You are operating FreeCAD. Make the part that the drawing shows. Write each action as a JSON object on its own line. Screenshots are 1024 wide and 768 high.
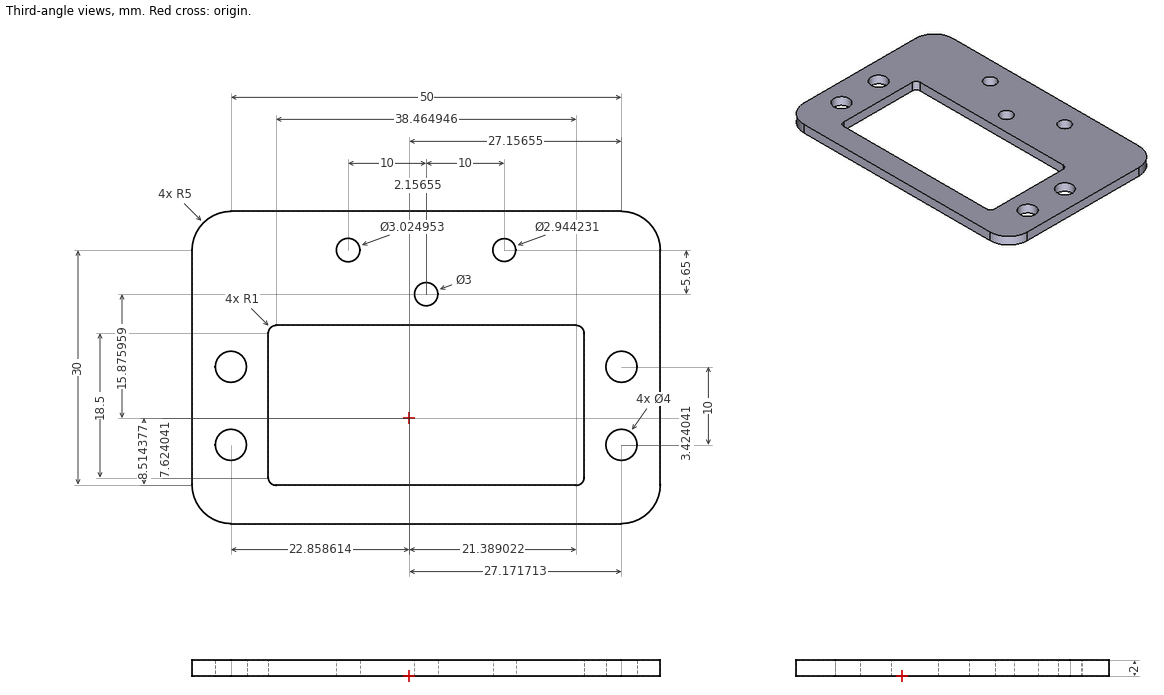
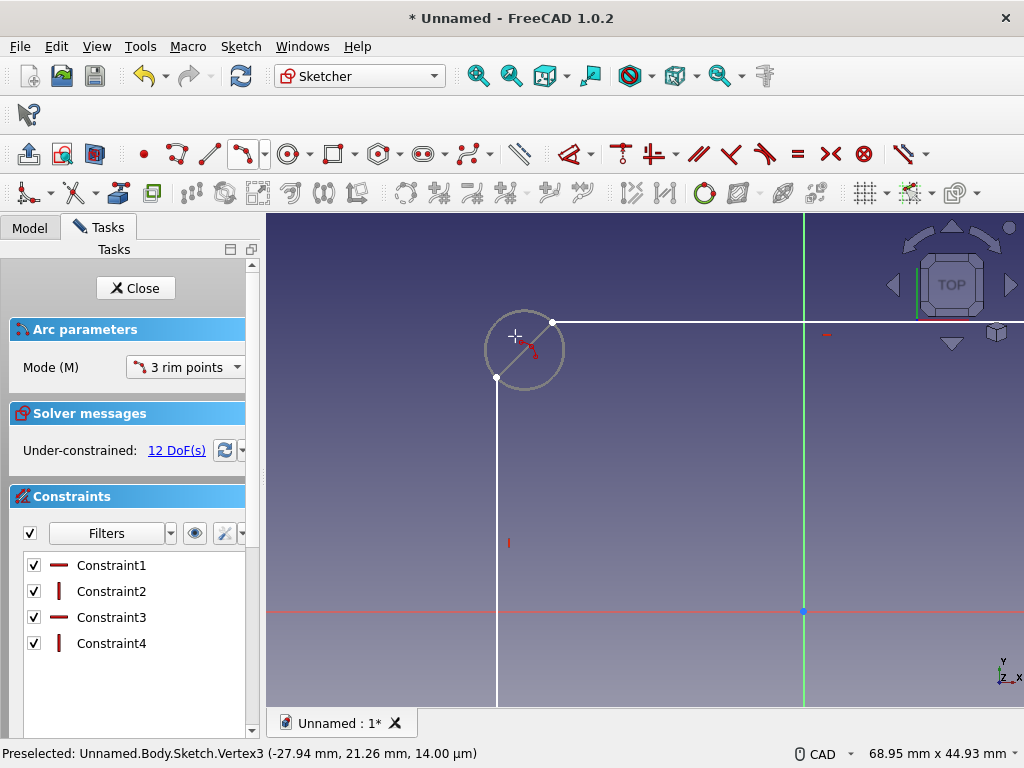
{"action": "left_click", "coordinate": [514, 337]}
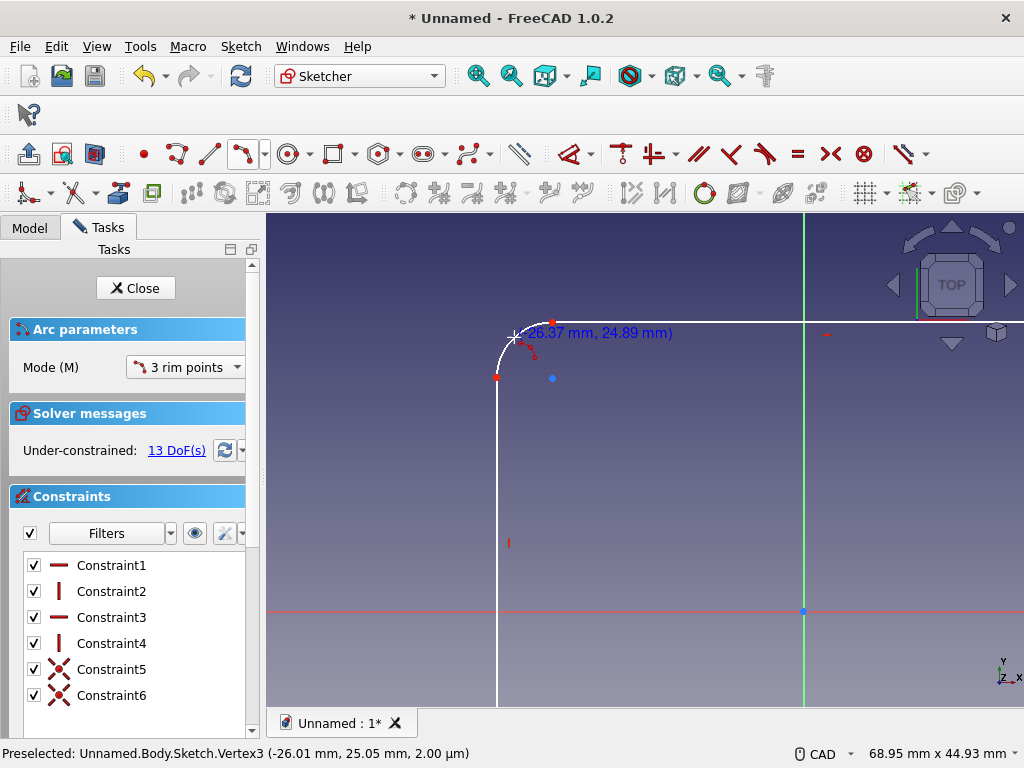
{"action": "scroll", "coordinate": [294, 362], "scroll_direction": "down", "scroll_amount": 3}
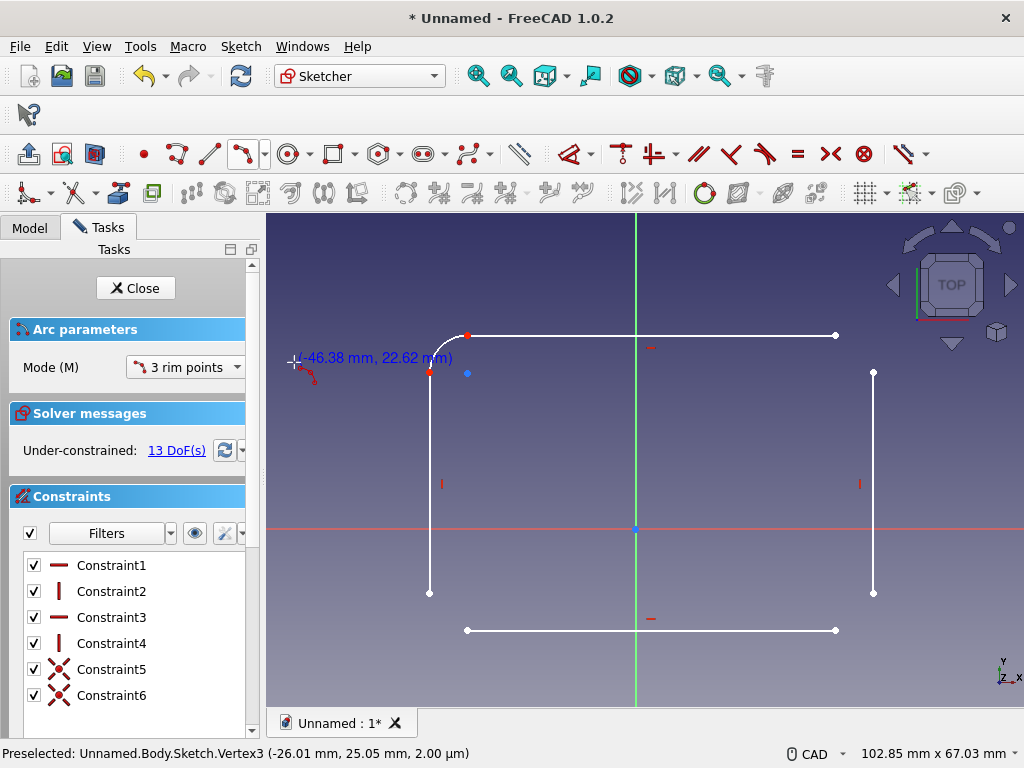
{"action": "left_click", "coordinate": [405, 552]}
{"action": "left_click", "coordinate": [436, 582]}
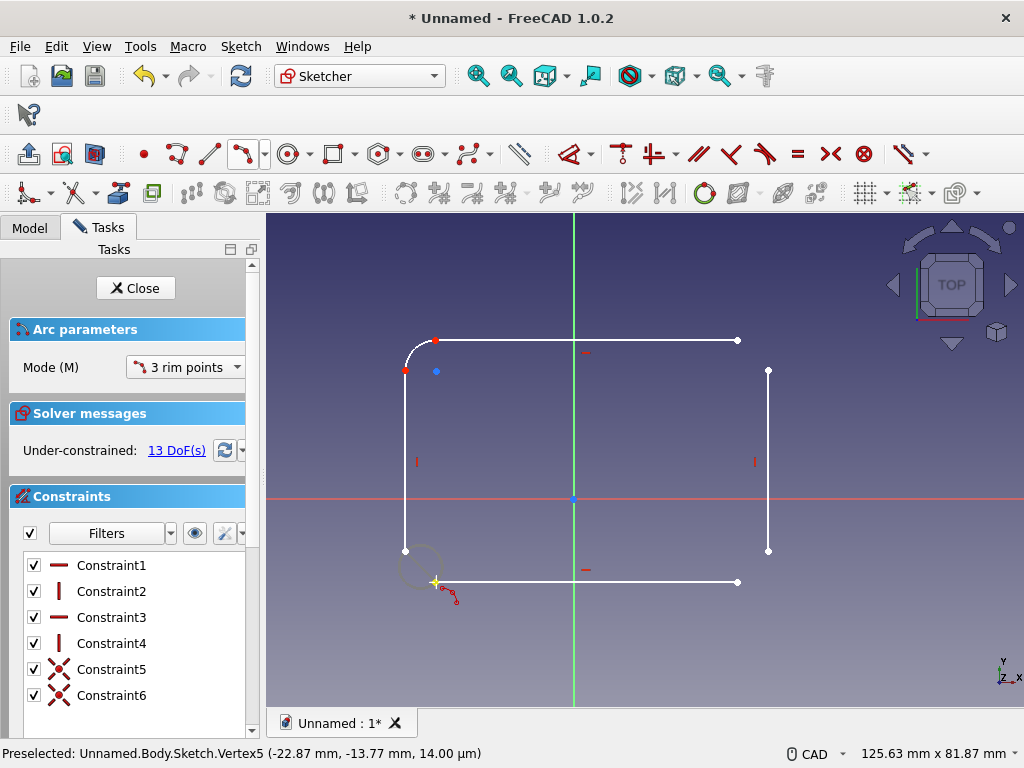
{"action": "scroll", "coordinate": [415, 572], "scroll_direction": "up", "scroll_amount": 3}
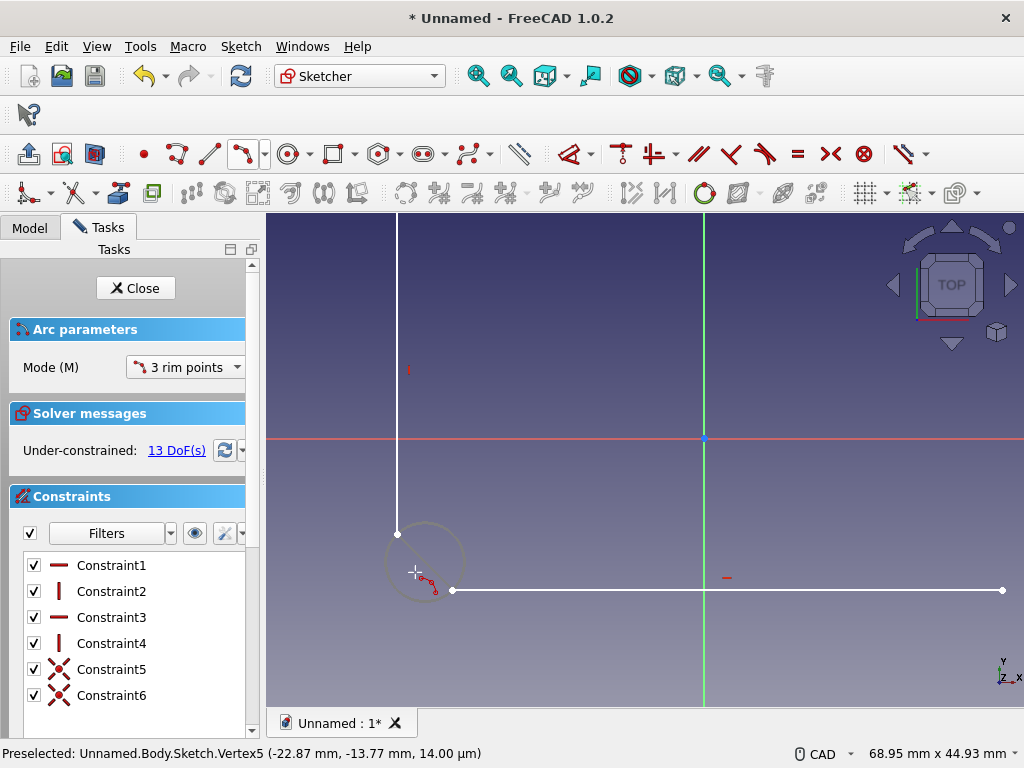
{"action": "left_click", "coordinate": [414, 571]}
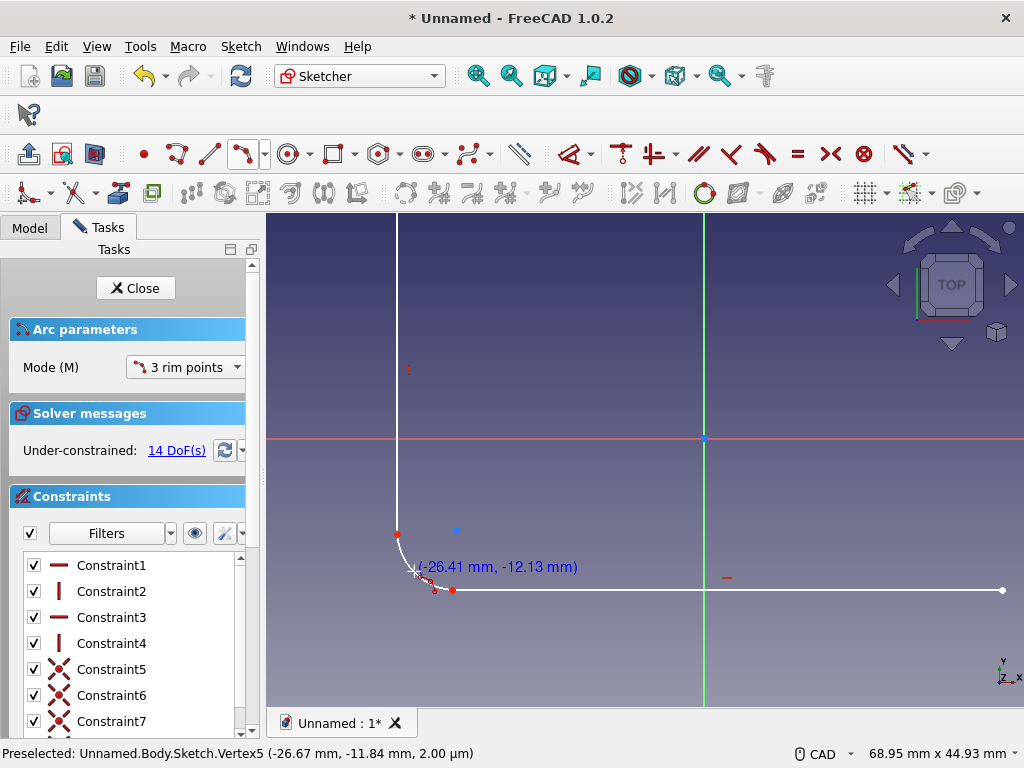
{"action": "scroll", "coordinate": [392, 573], "scroll_direction": "down", "scroll_amount": 3}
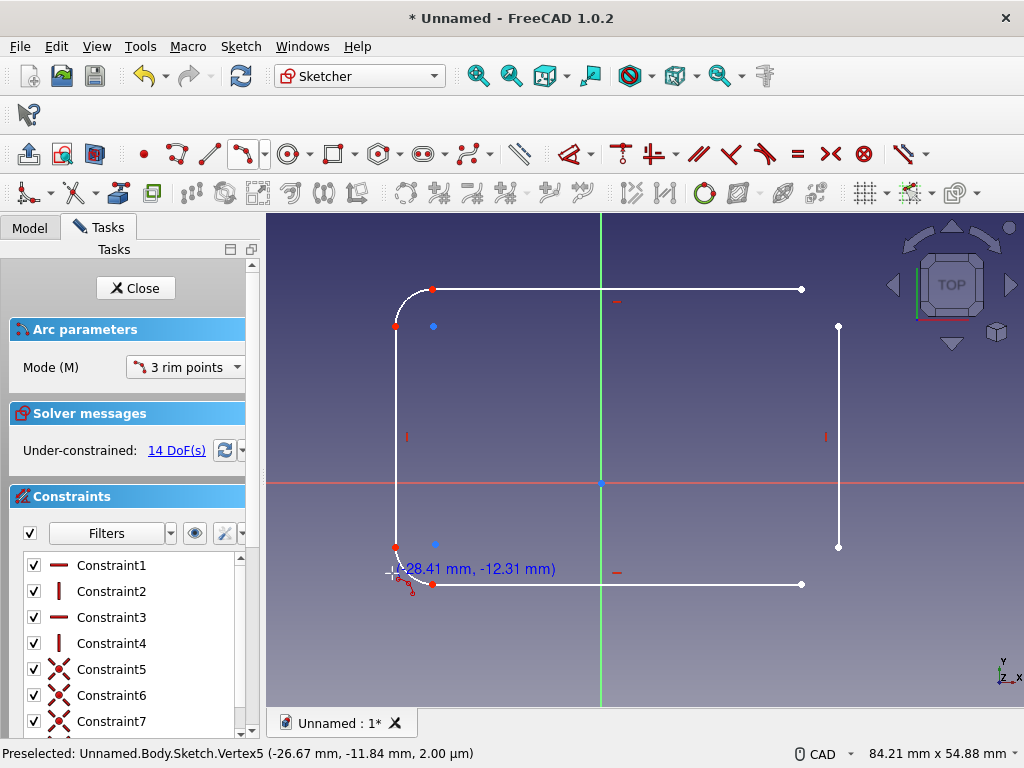
{"action": "left_click", "coordinate": [727, 583]}
{"action": "left_click", "coordinate": [758, 552]}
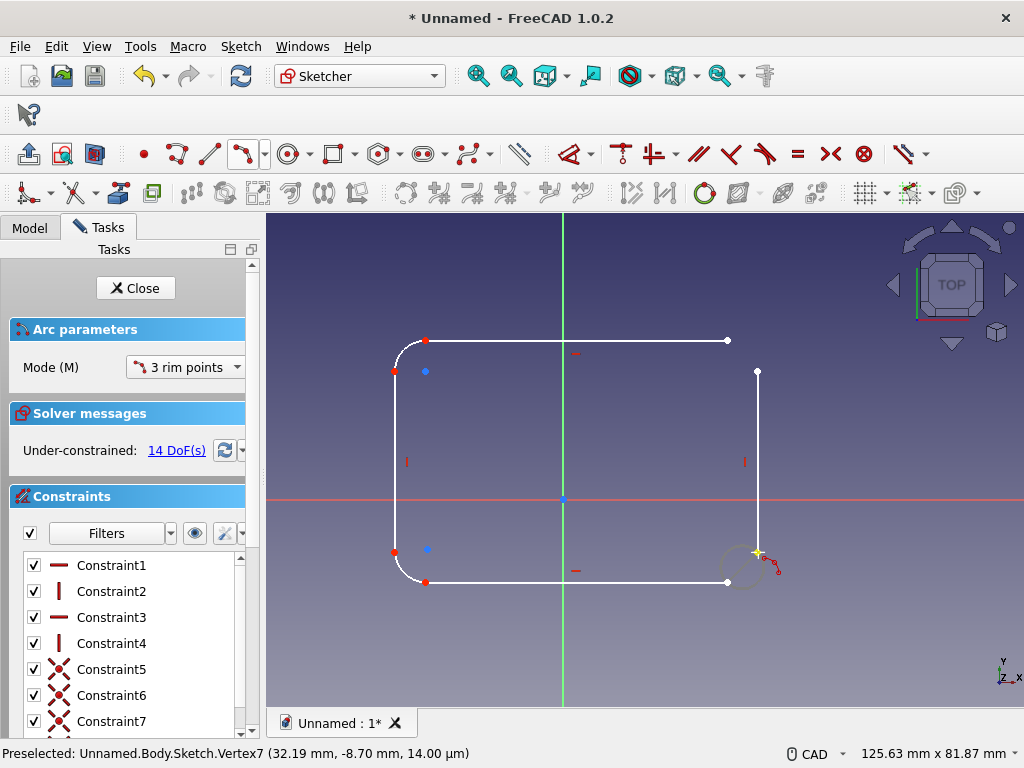
{"action": "scroll", "coordinate": [749, 572], "scroll_direction": "up", "scroll_amount": 3}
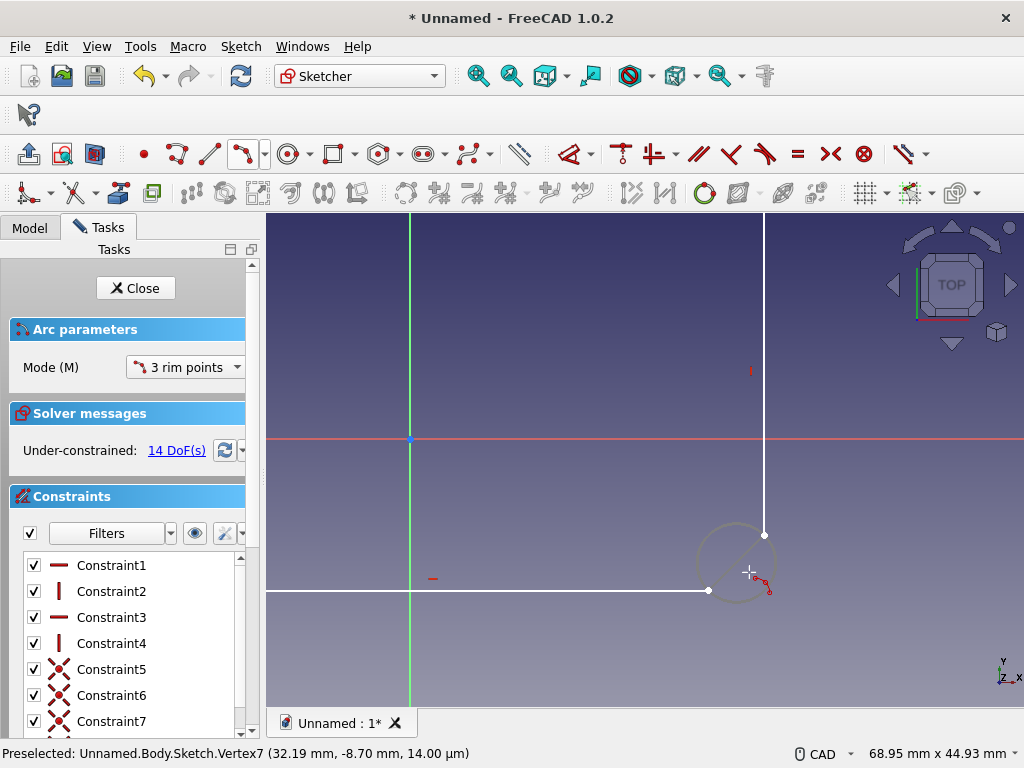
{"action": "left_click", "coordinate": [748, 572]}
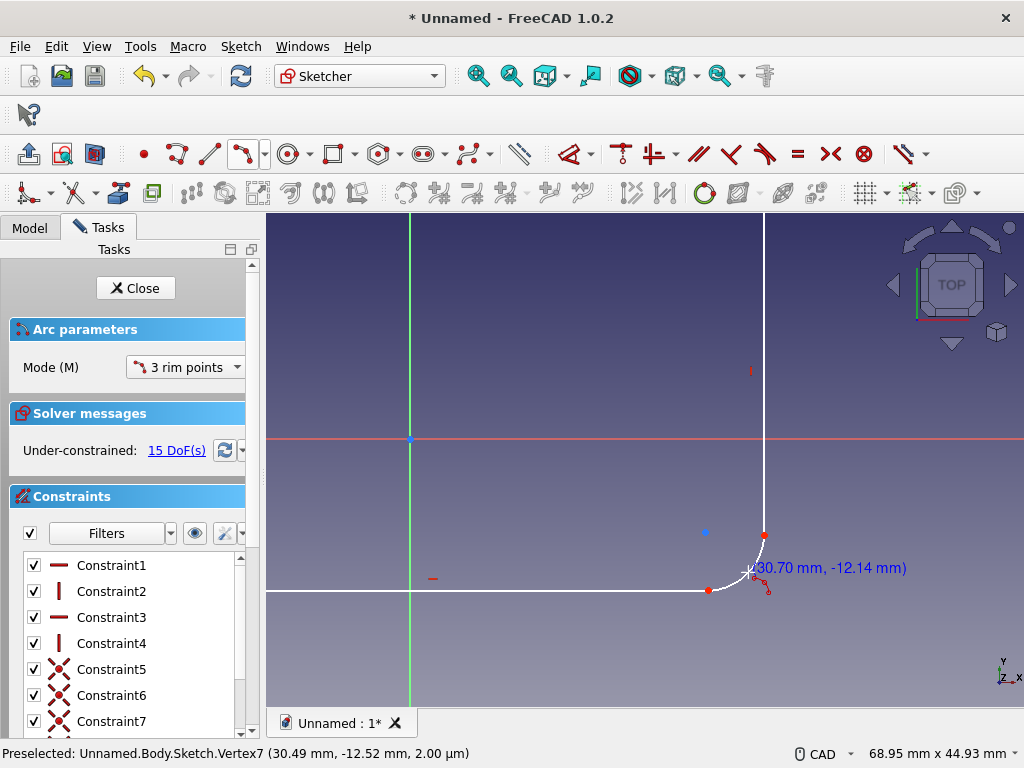
{"action": "scroll", "coordinate": [750, 572], "scroll_direction": "down", "scroll_amount": 3}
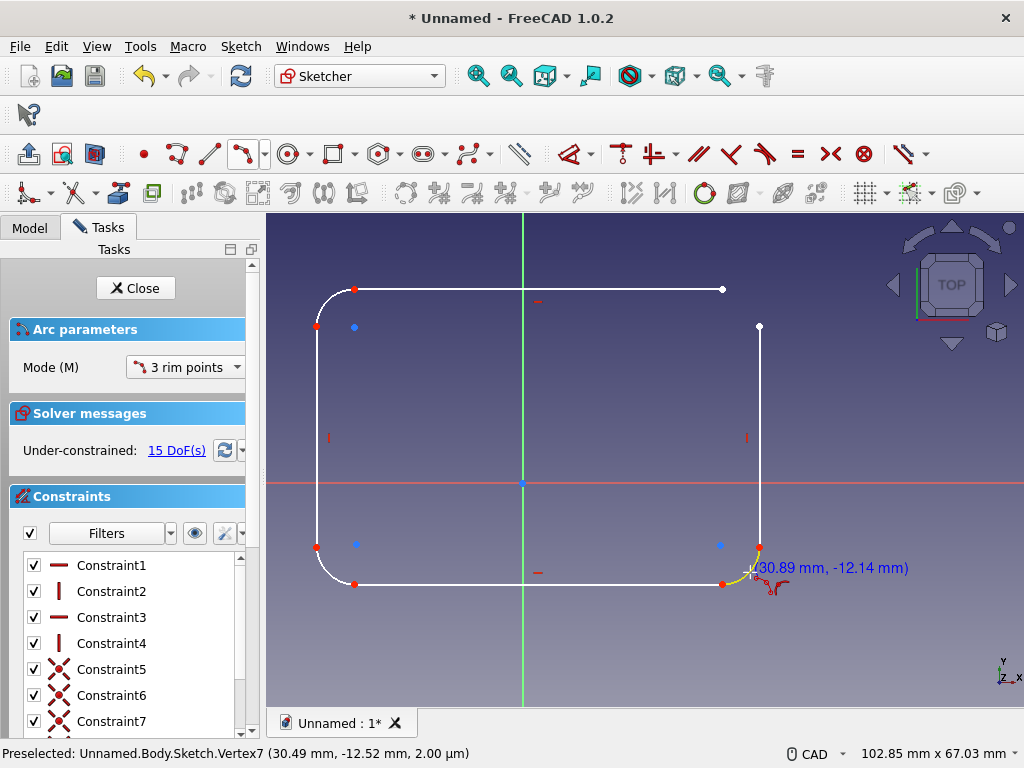
{"action": "left_click", "coordinate": [758, 371]}
{"action": "left_click", "coordinate": [728, 341]}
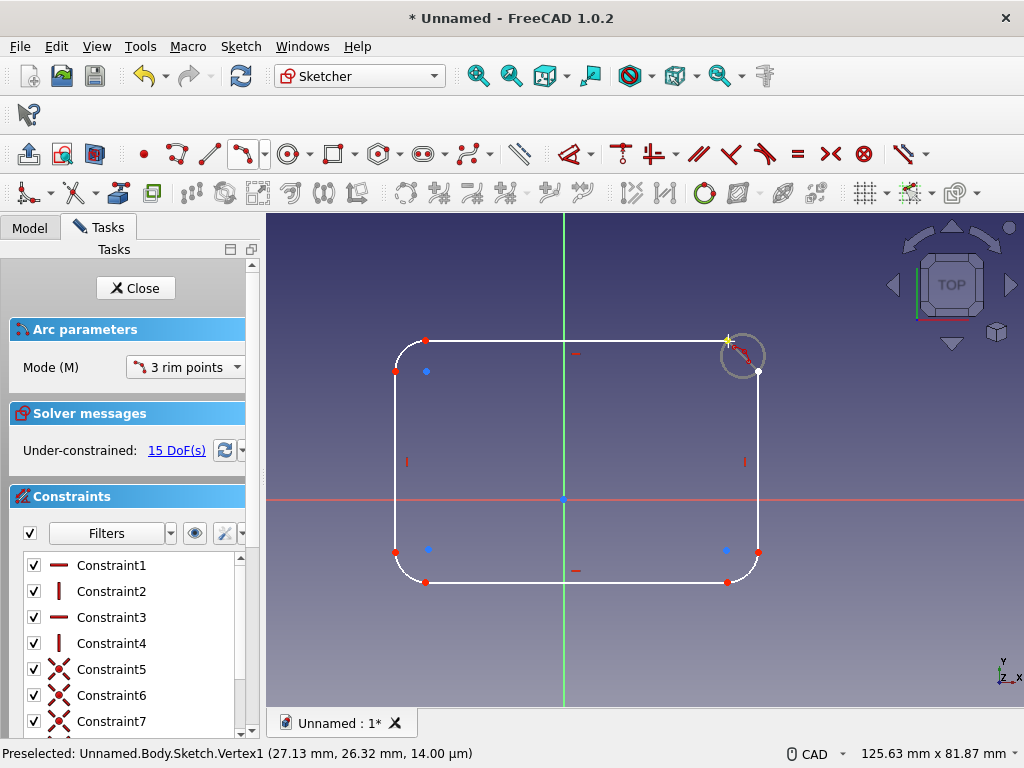
{"action": "scroll", "coordinate": [749, 349], "scroll_direction": "up", "scroll_amount": 3}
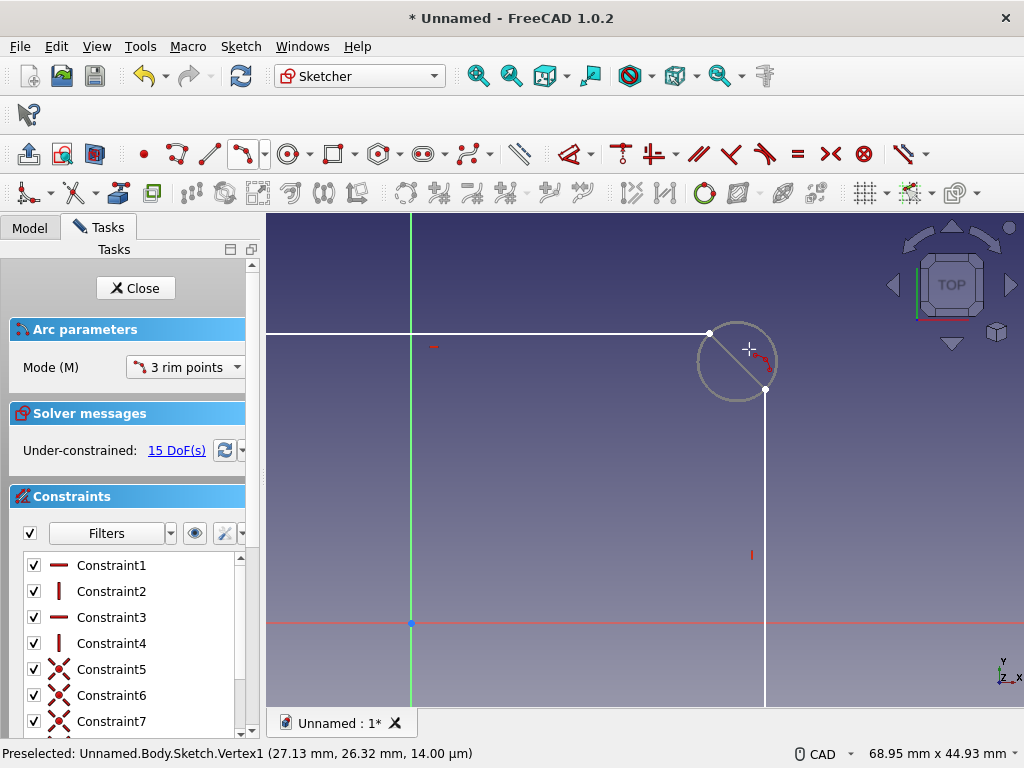
{"action": "left_click", "coordinate": [749, 348]}
{"action": "key", "text": "Escape"}